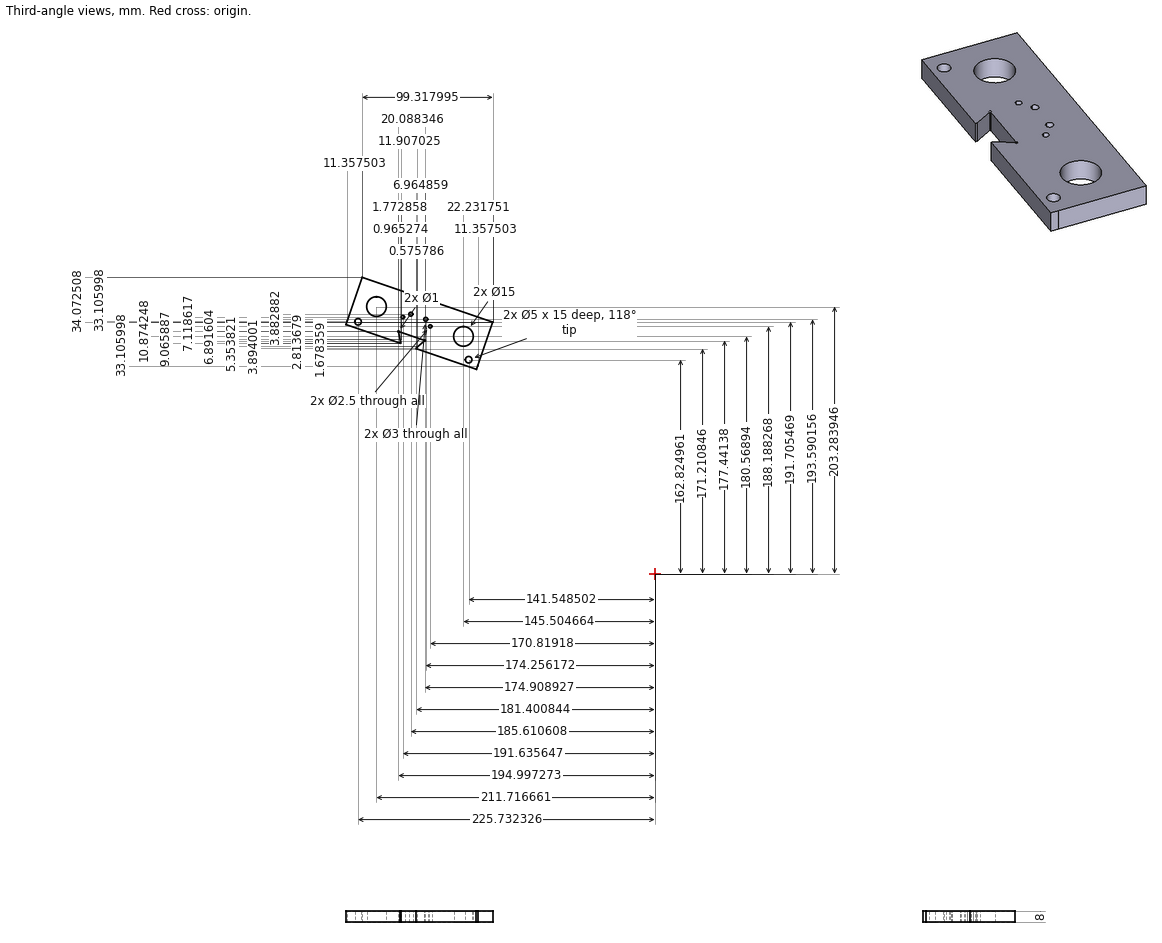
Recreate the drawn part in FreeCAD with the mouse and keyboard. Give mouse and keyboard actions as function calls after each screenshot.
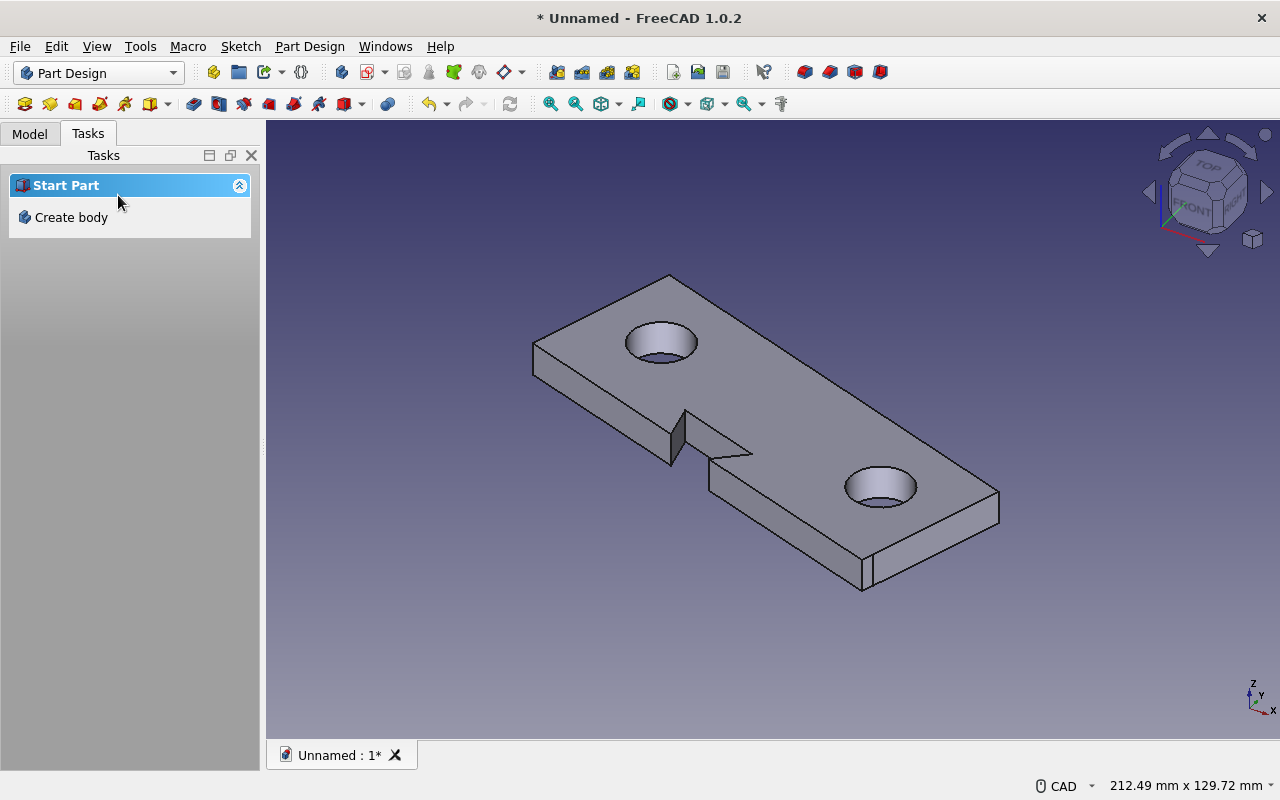
click(832, 438)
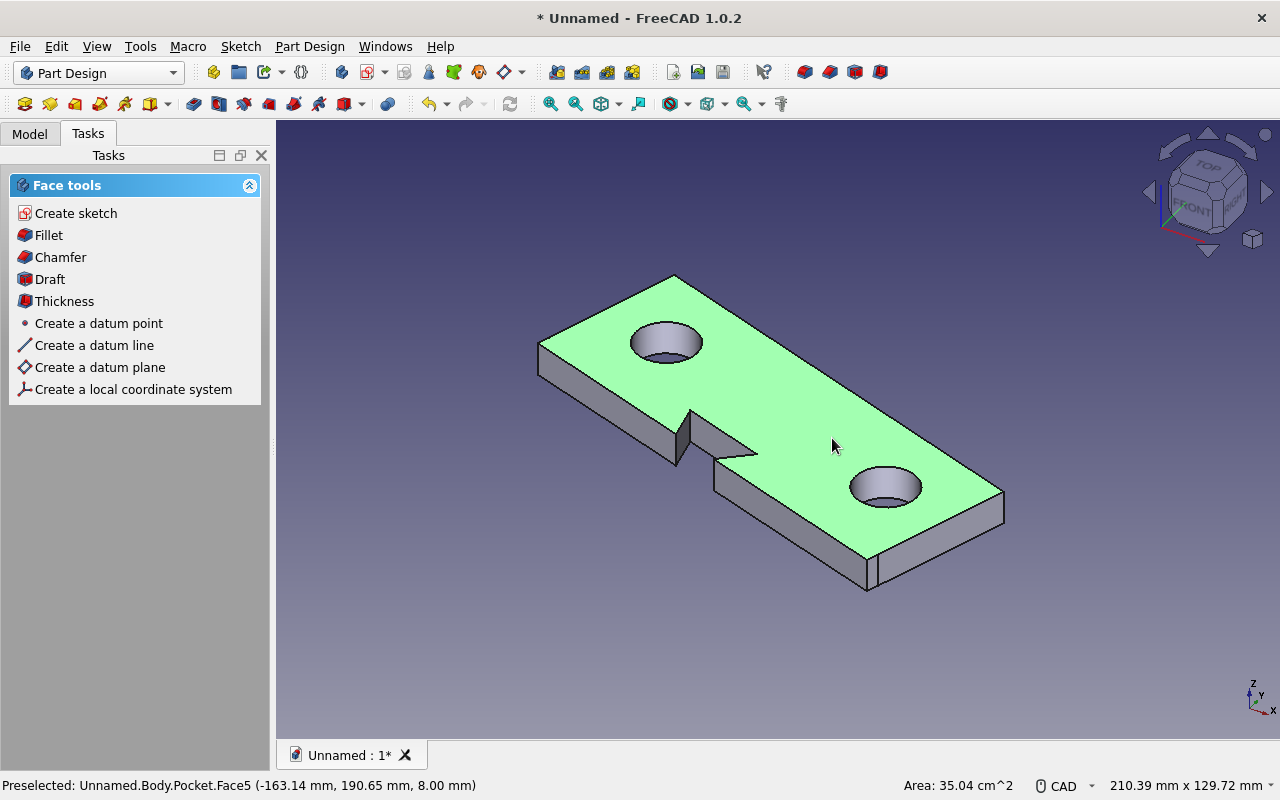
click(366, 72)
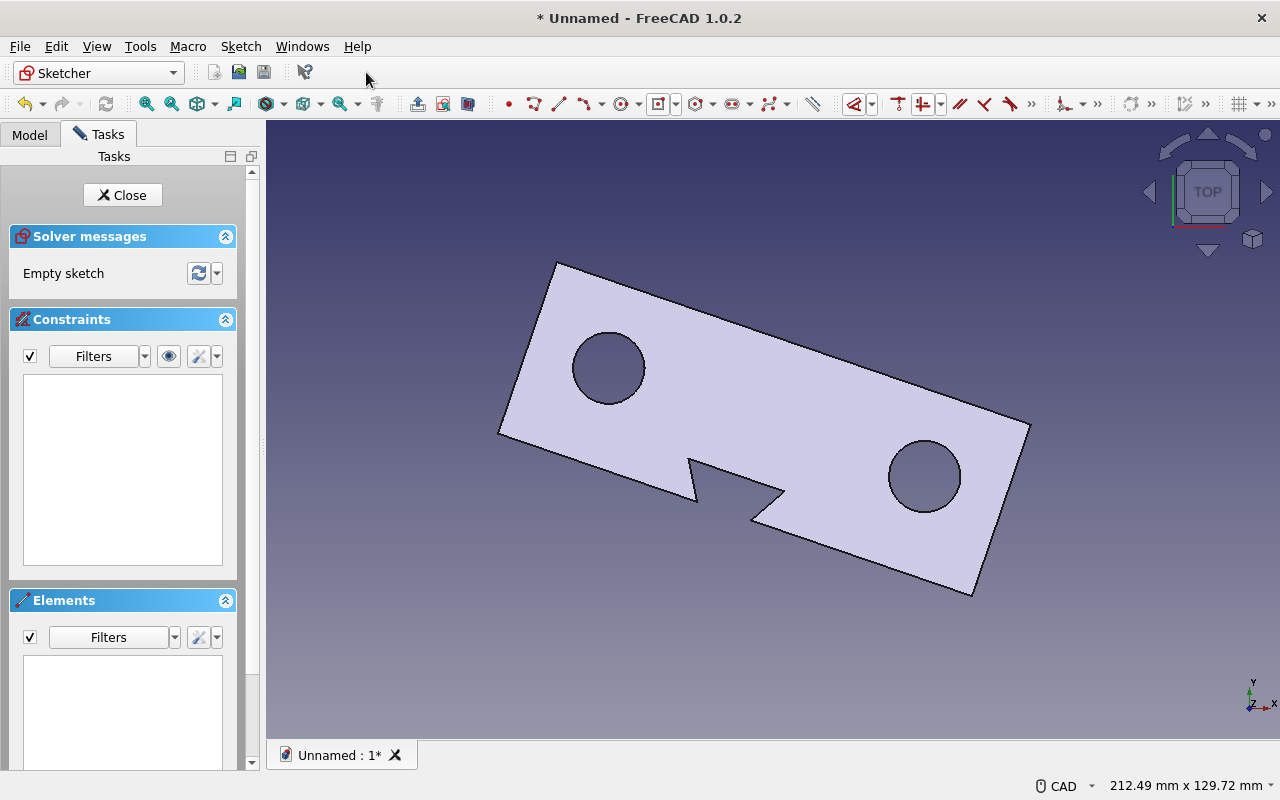
scroll(820, 620, up, 2)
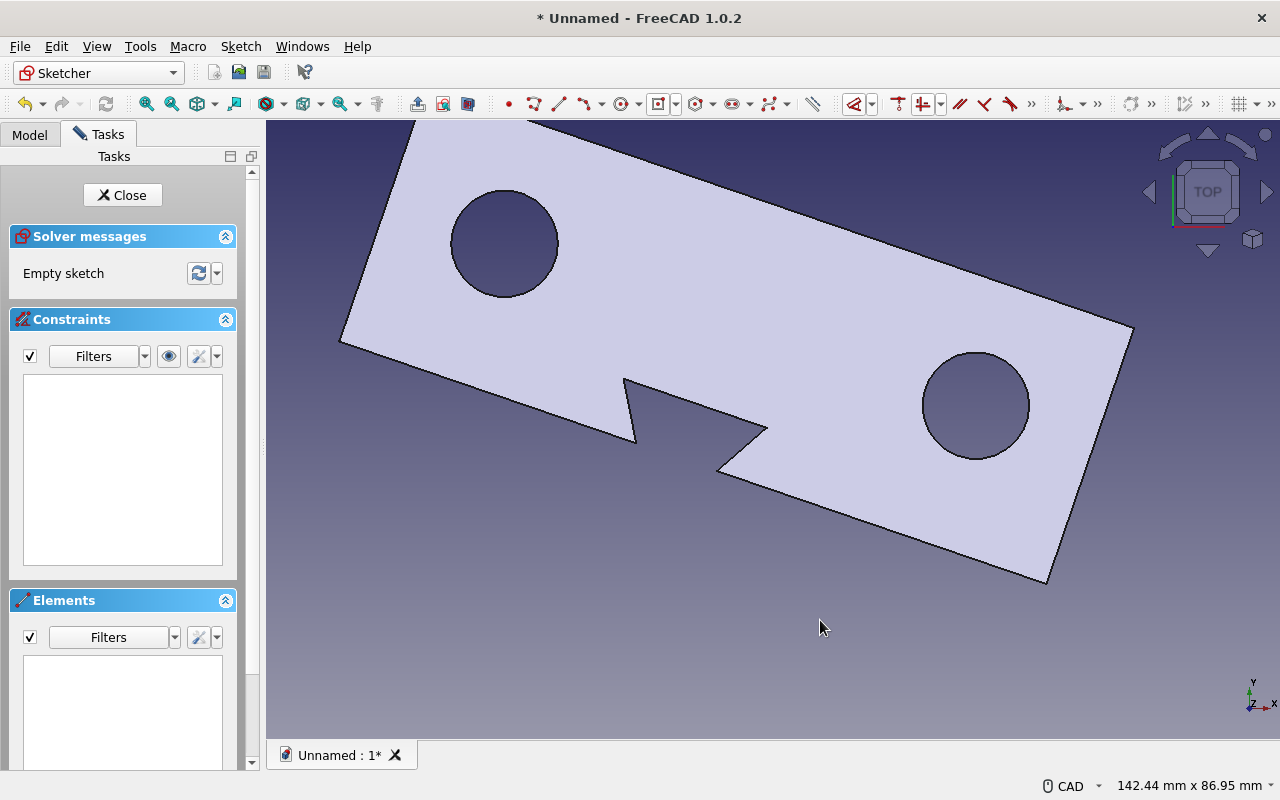
key(g)
key(c)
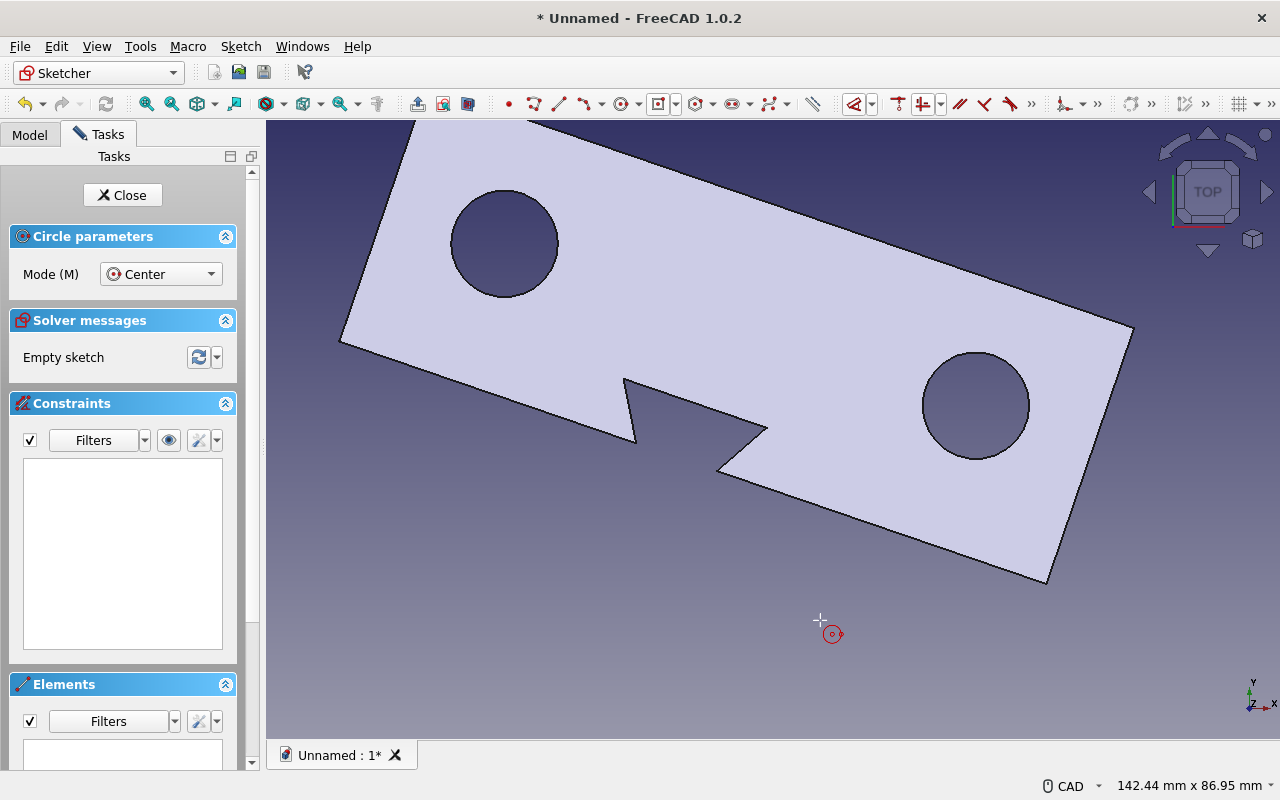
scroll(1004, 532, up, 2)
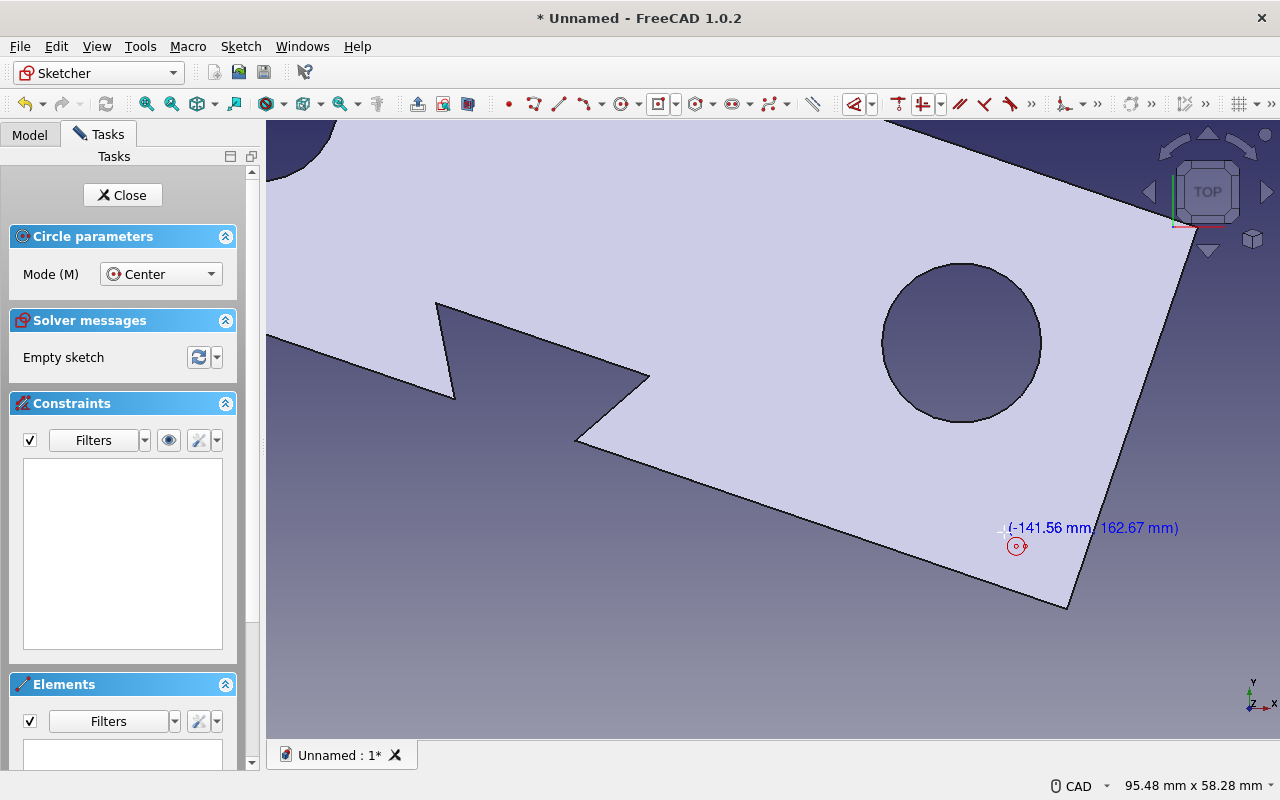
click(1004, 531)
click(1023, 513)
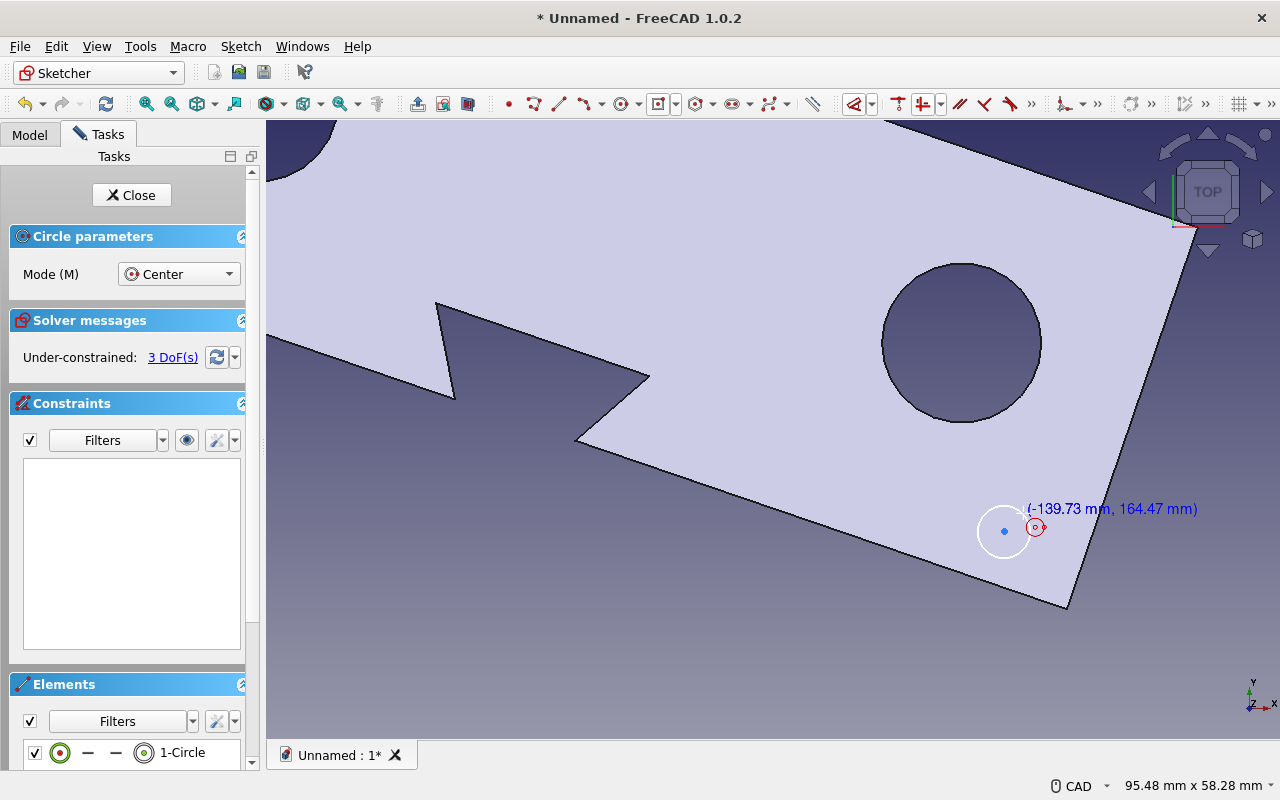
scroll(1005, 534, down, 2)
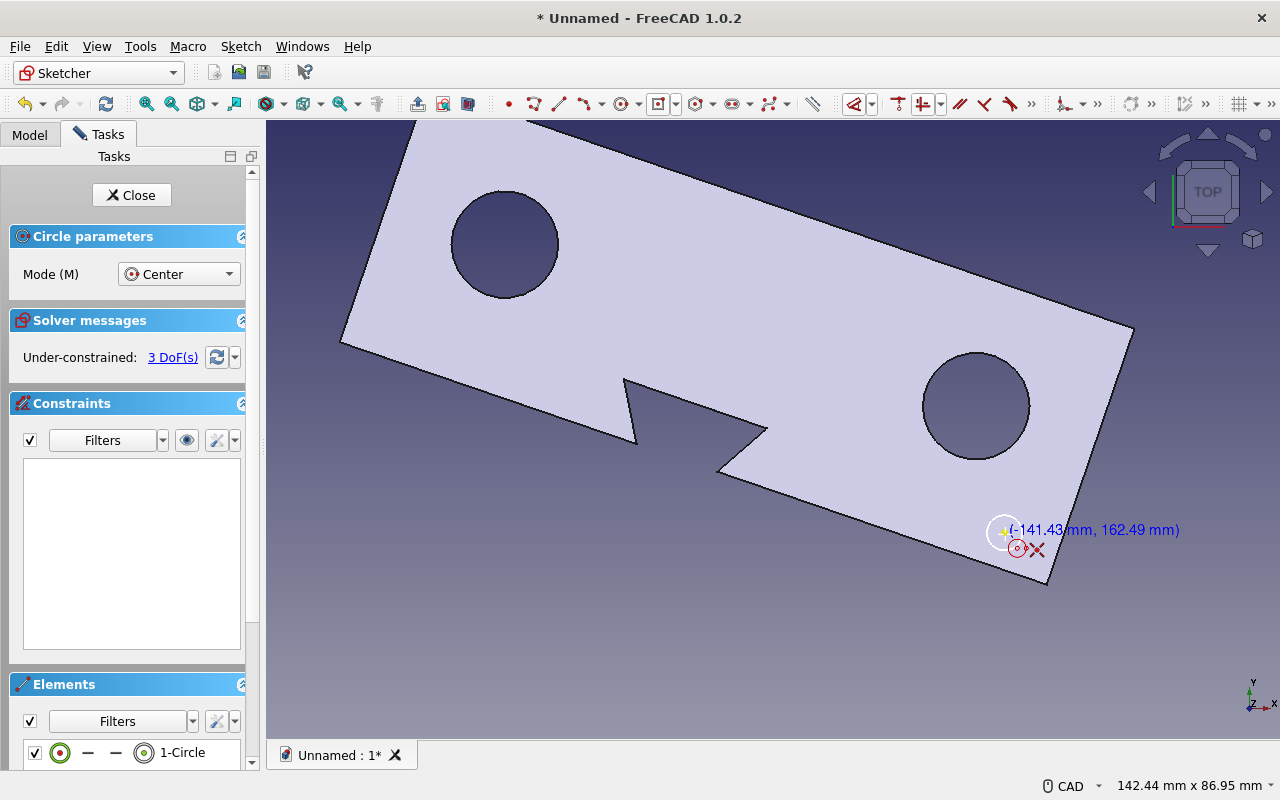
scroll(405, 327, up, 2)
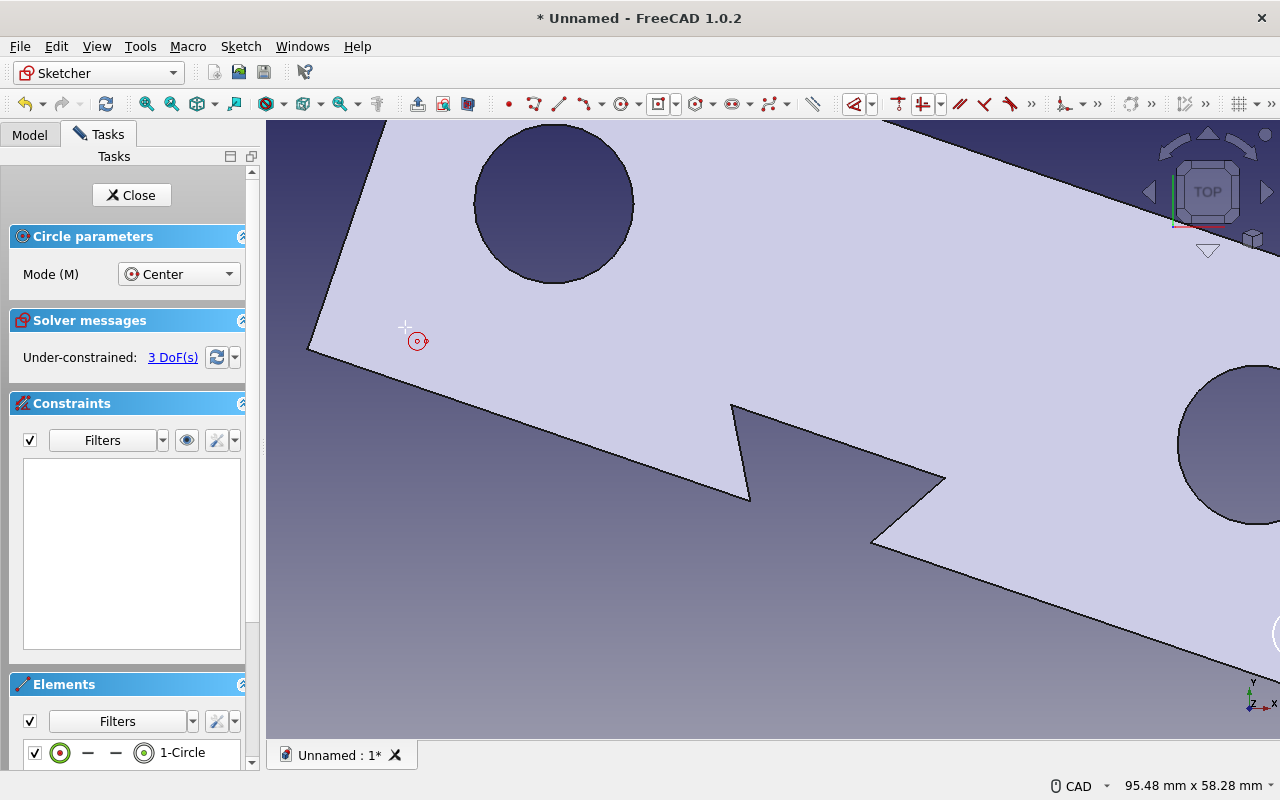
click(405, 327)
click(424, 308)
key(Escape)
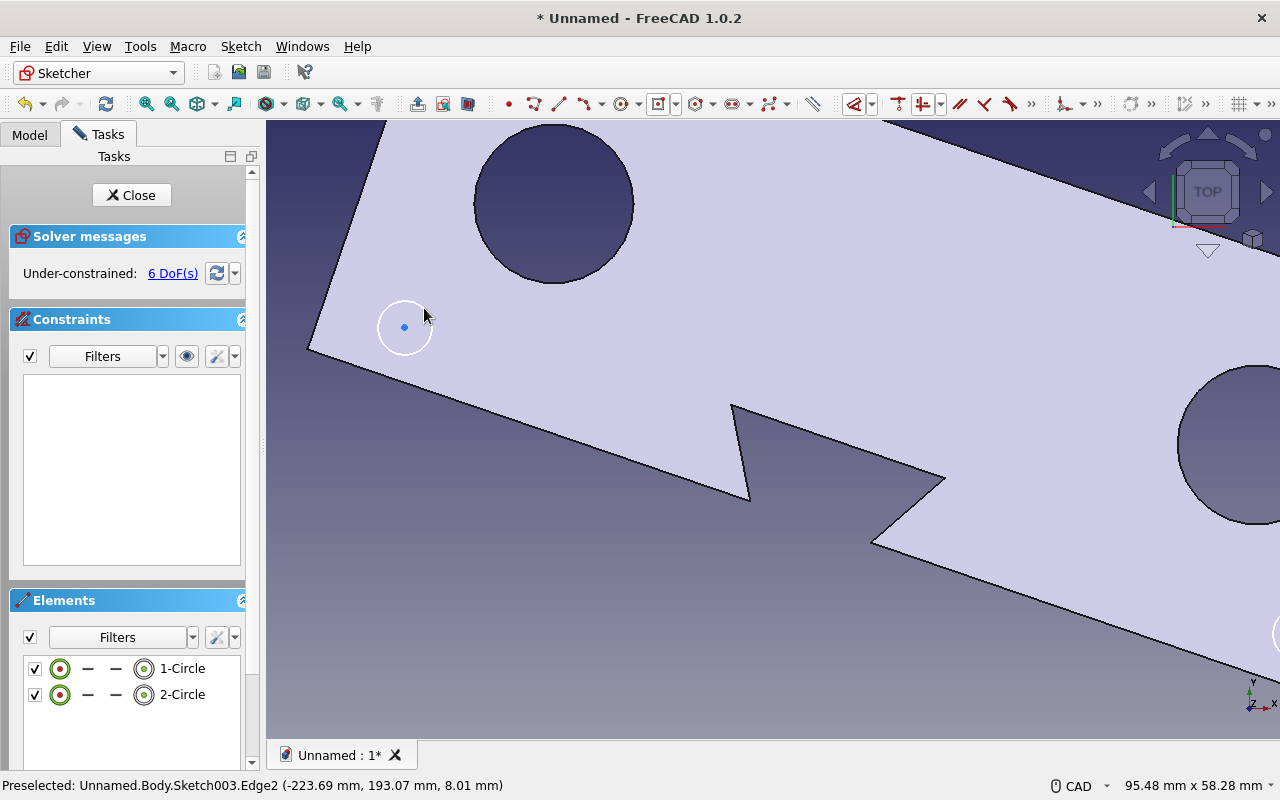
scroll(404, 327, down, 2)